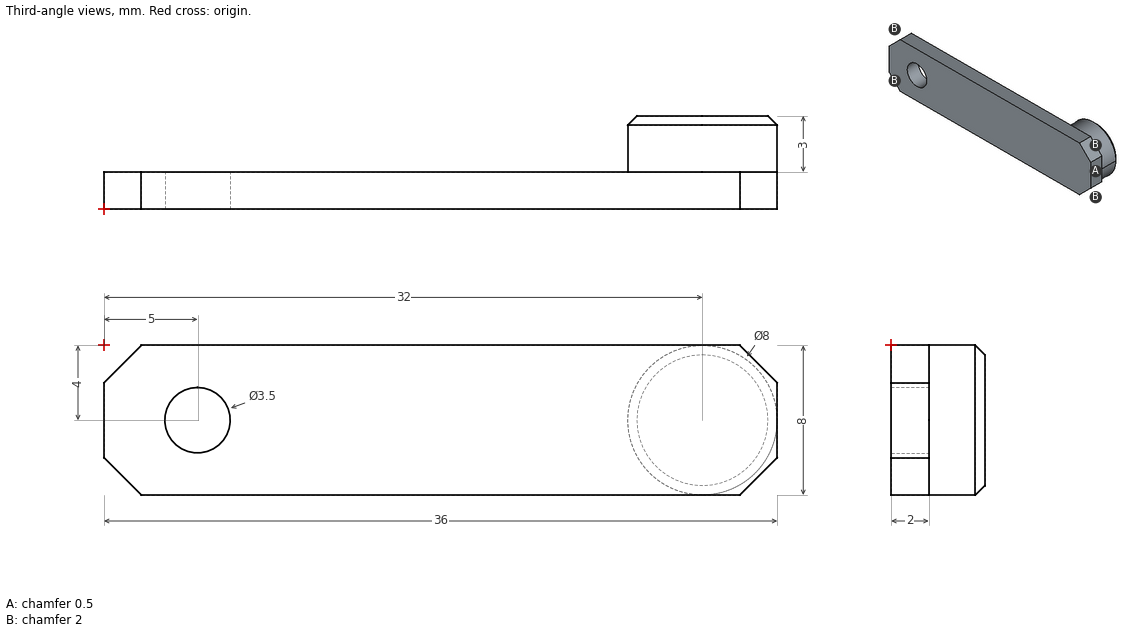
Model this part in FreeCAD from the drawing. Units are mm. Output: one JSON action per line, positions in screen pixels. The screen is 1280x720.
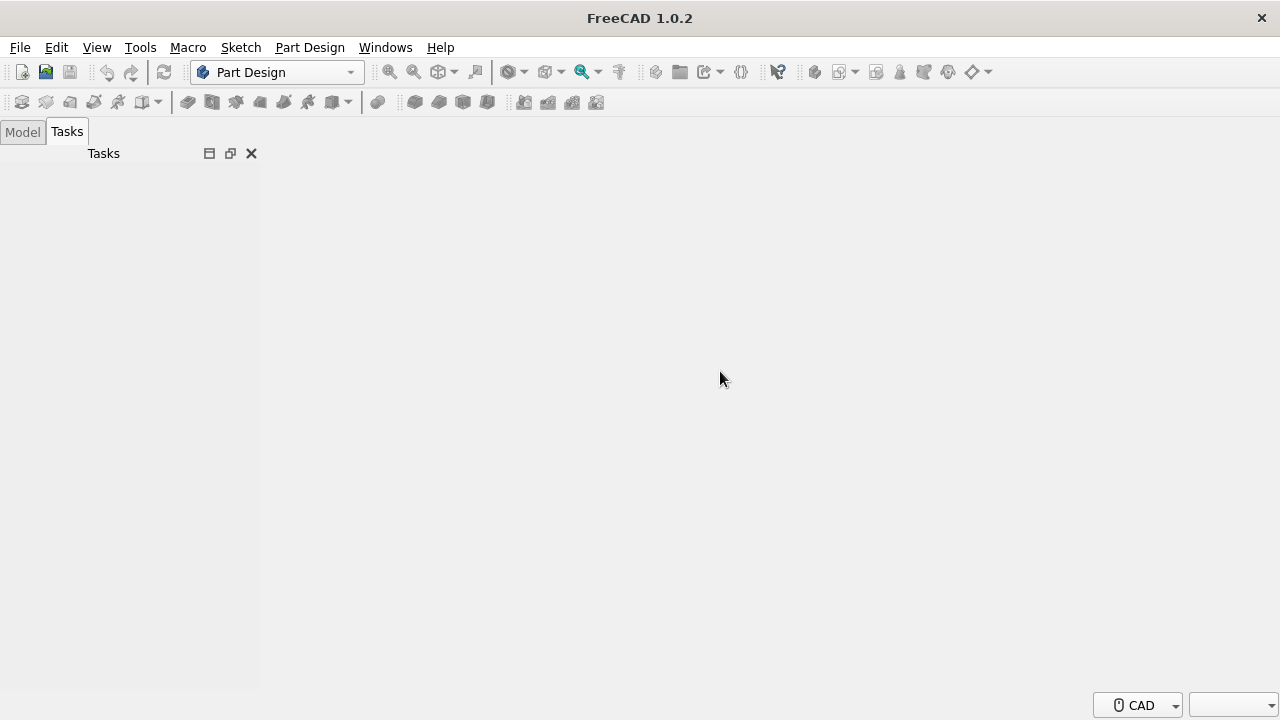
{"action": "key", "text": "ctrl+n"}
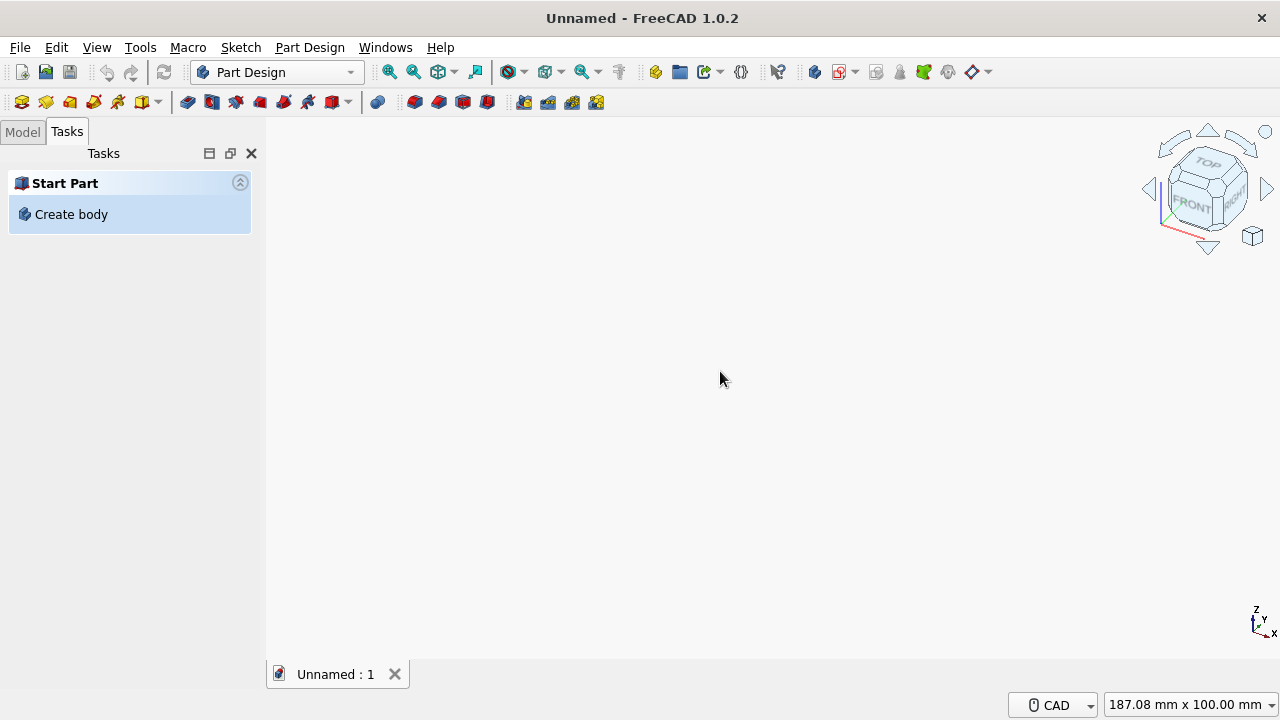
{"action": "left_click", "coordinate": [840, 72]}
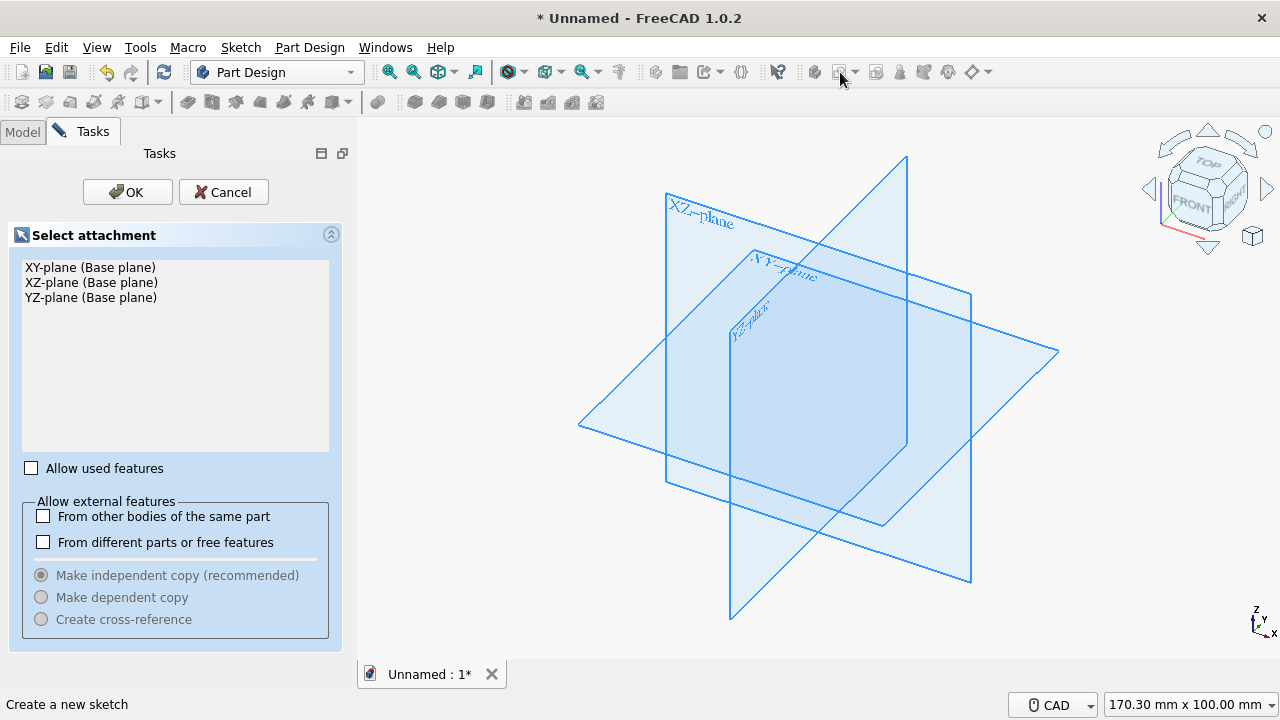
{"action": "left_click", "coordinate": [82, 282]}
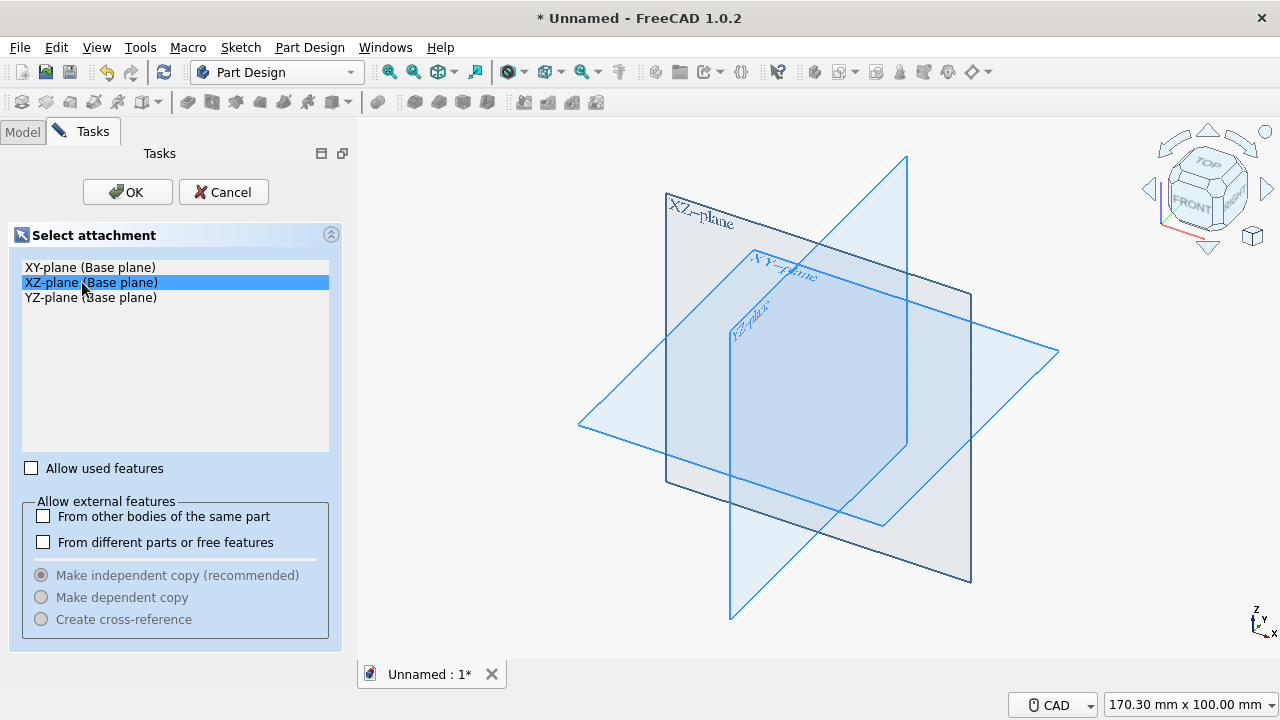
{"action": "left_click", "coordinate": [128, 192]}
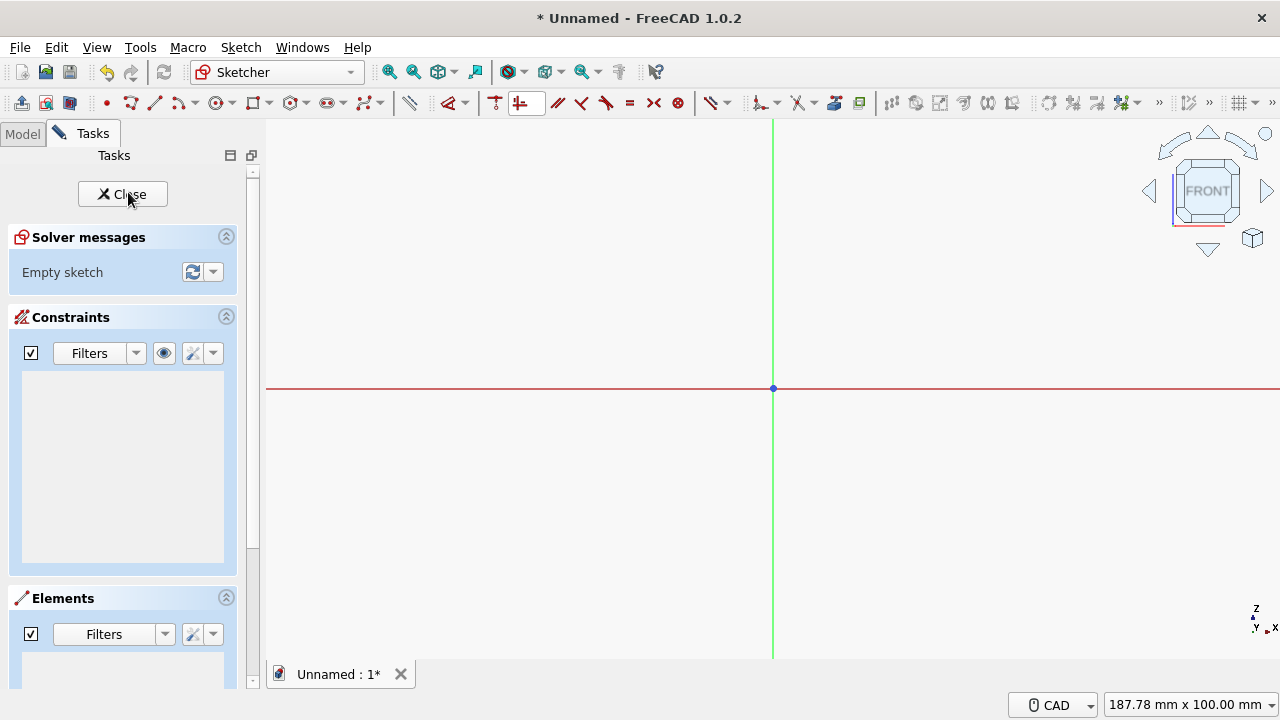
{"action": "scroll", "coordinate": [967, 423], "scroll_direction": "up", "scroll_amount": 5}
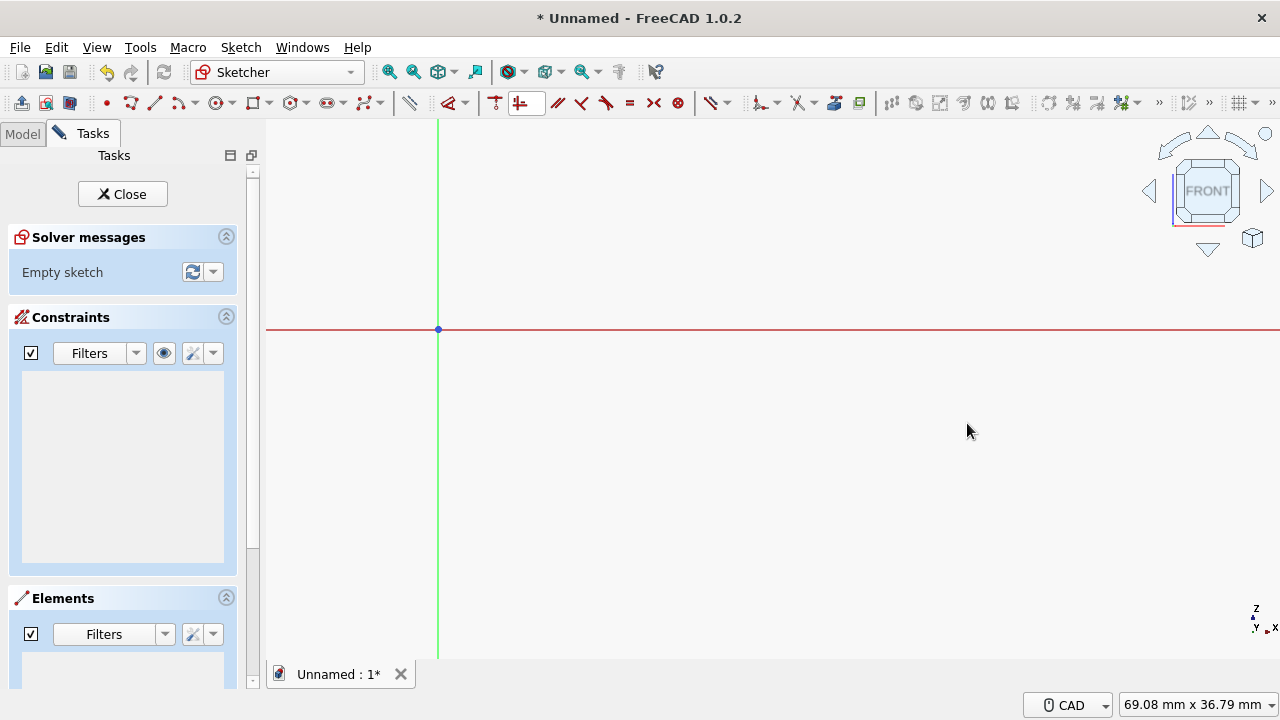
{"action": "left_click", "coordinate": [254, 104]}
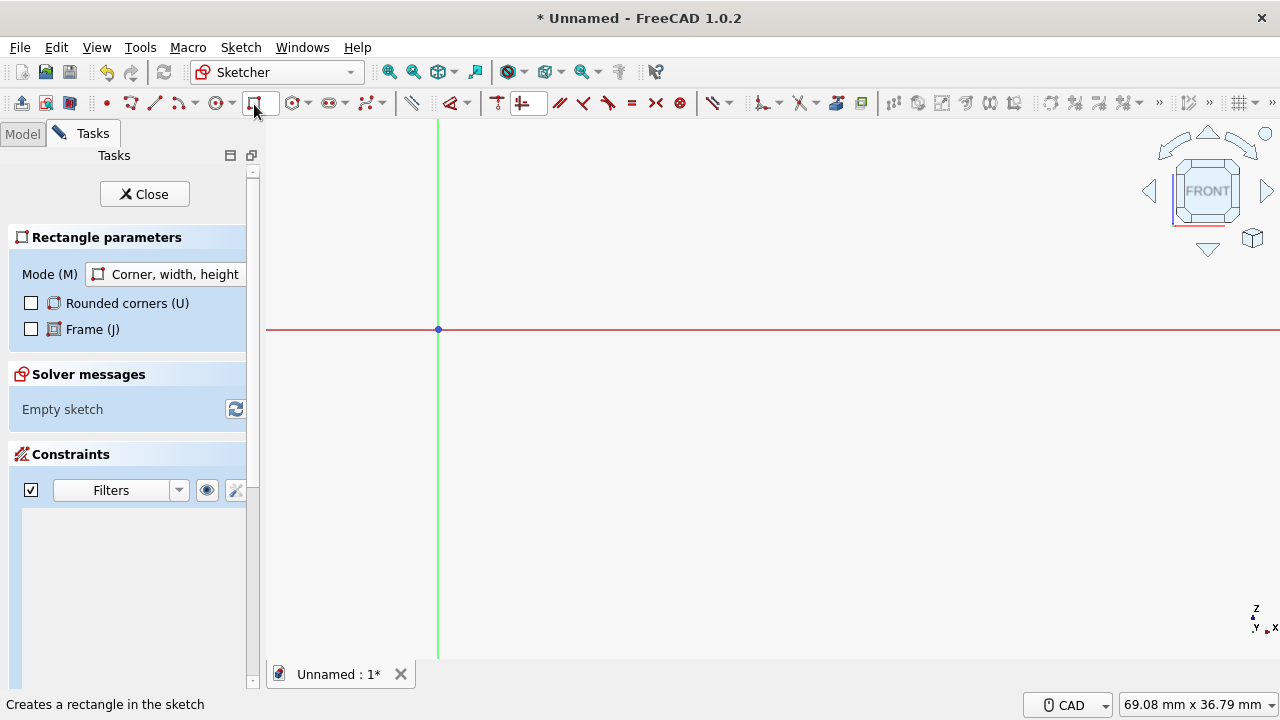
{"action": "left_click", "coordinate": [438, 330]}
{"action": "mouse_move", "coordinate": [967, 447]}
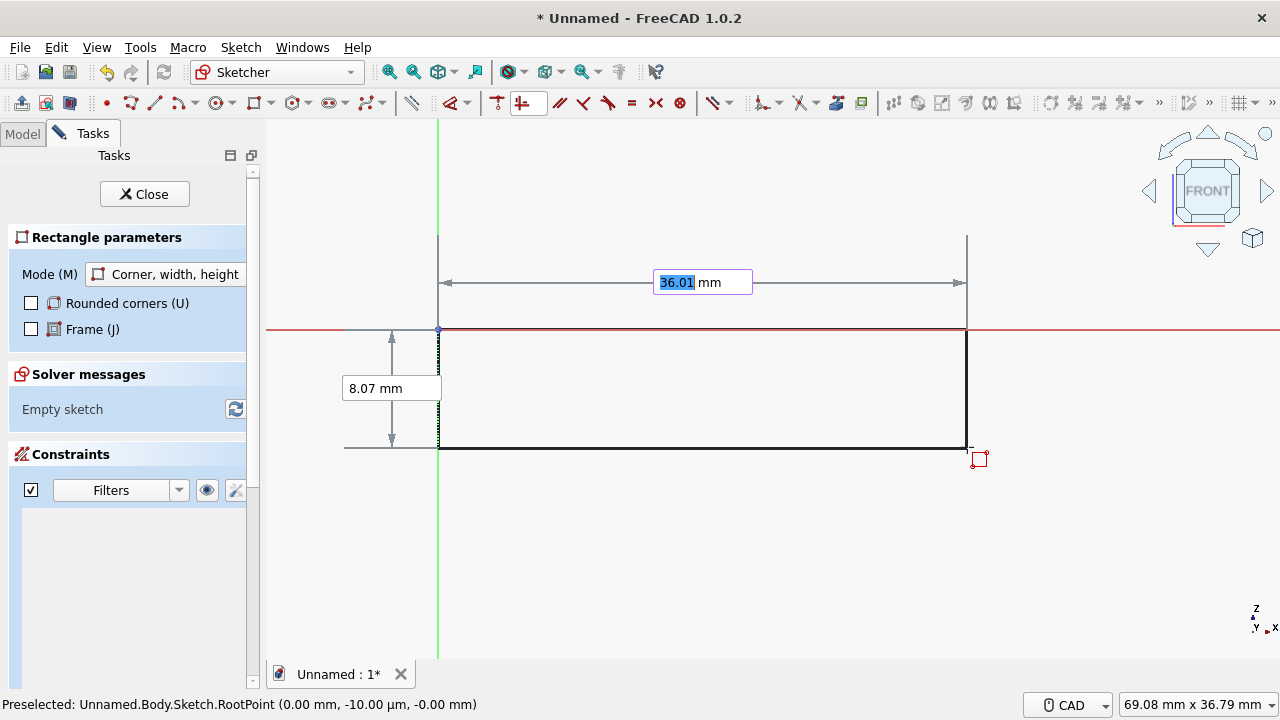
{"action": "type", "text": "36"}
{"action": "key", "text": "Tab"}
{"action": "type", "text": "8"}
{"action": "key", "text": "Return"}
{"action": "key", "text": "Escape"}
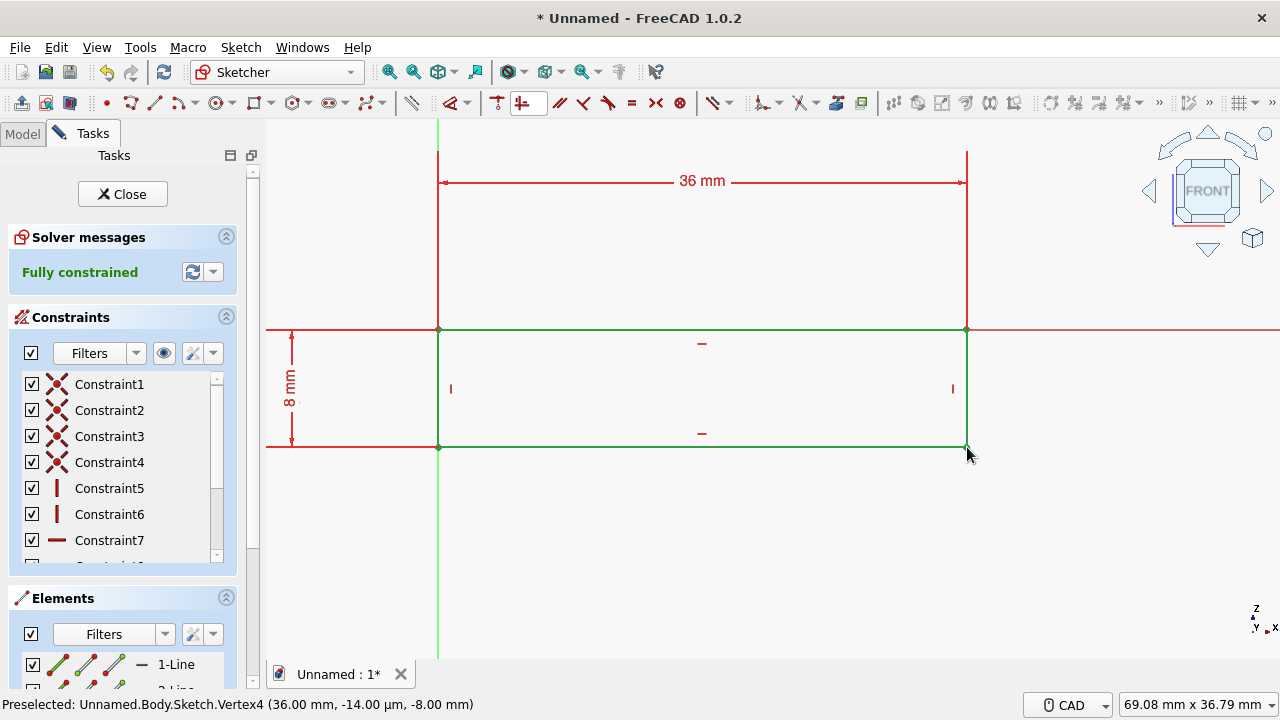
{"action": "left_click", "coordinate": [123, 194]}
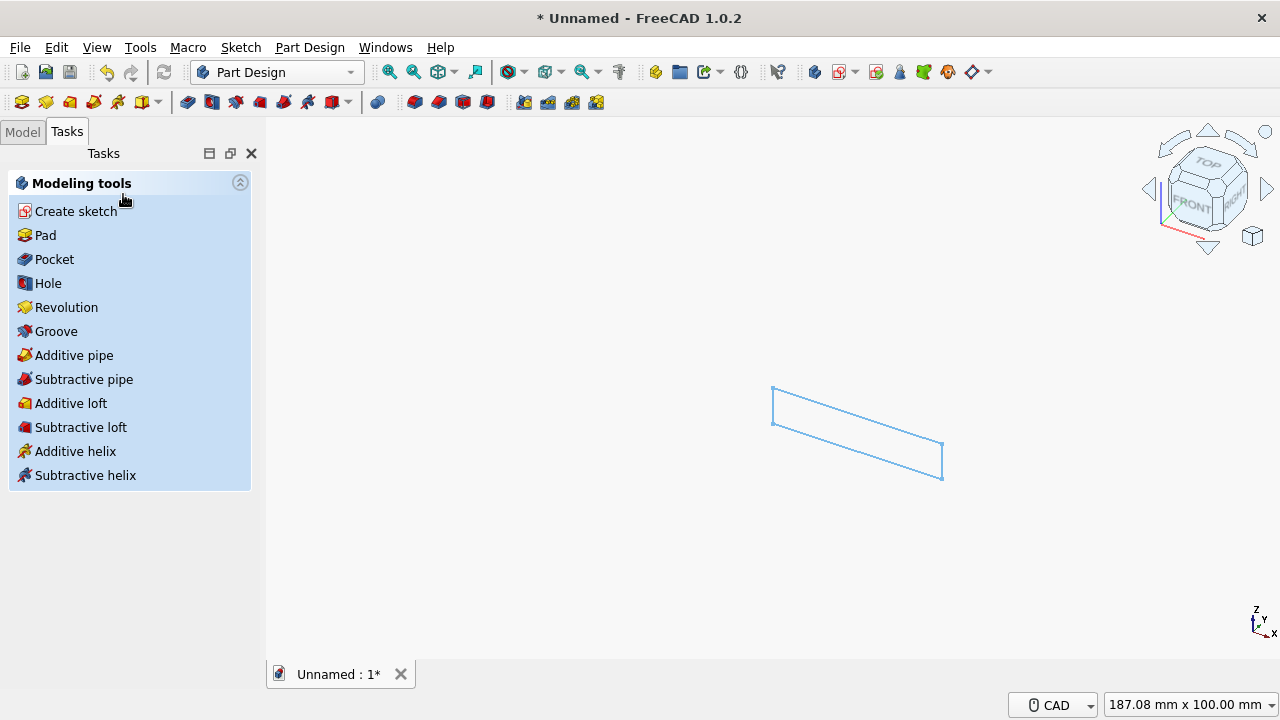
{"action": "left_click", "coordinate": [22, 102]}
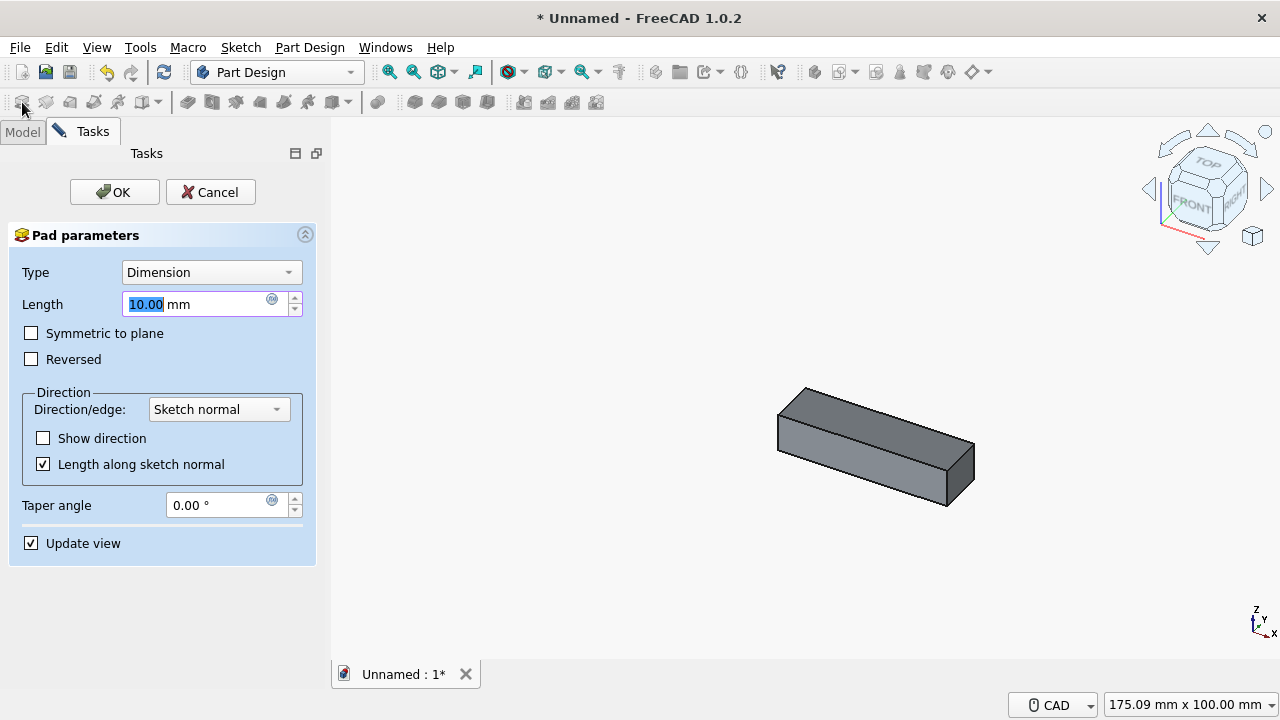
{"action": "type", "text": "2"}
{"action": "key", "text": "Tab"}